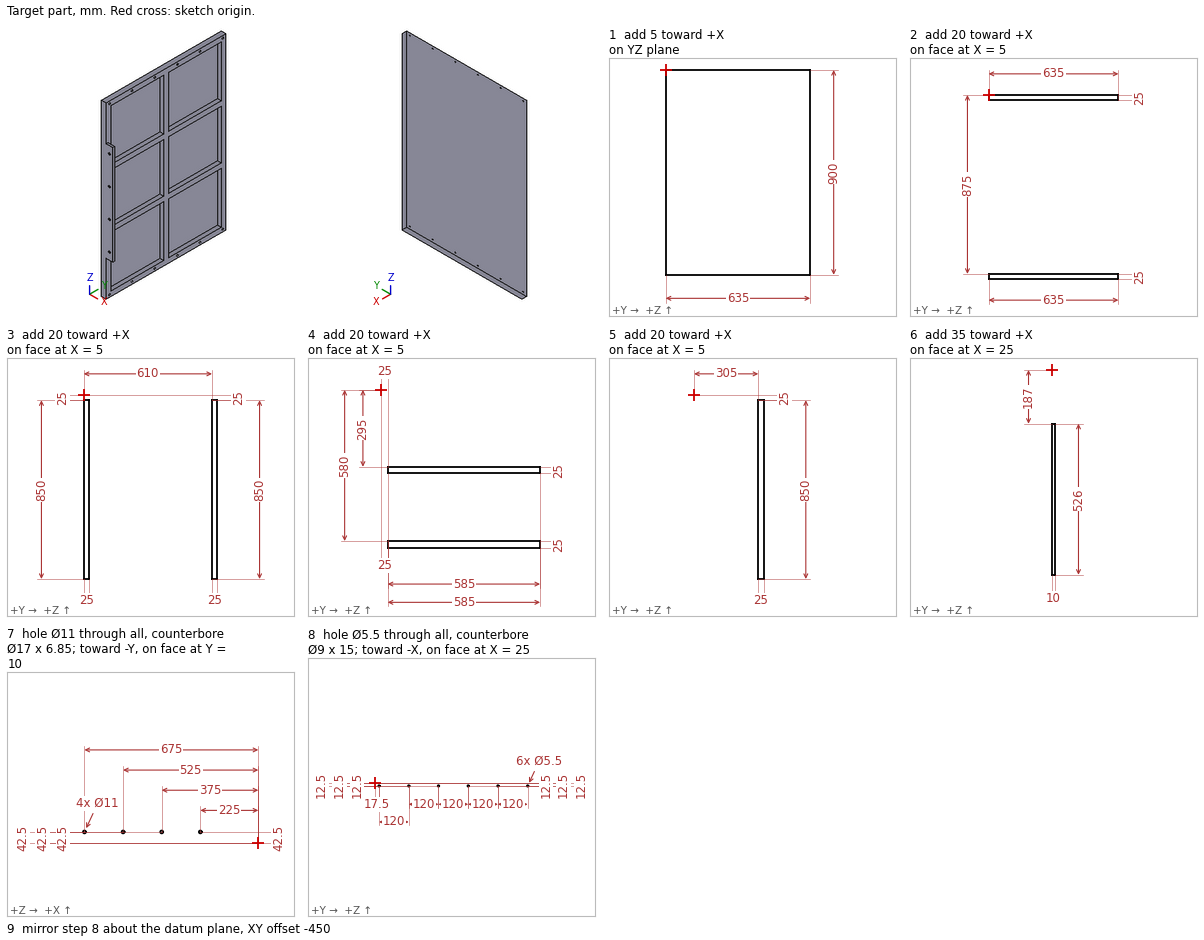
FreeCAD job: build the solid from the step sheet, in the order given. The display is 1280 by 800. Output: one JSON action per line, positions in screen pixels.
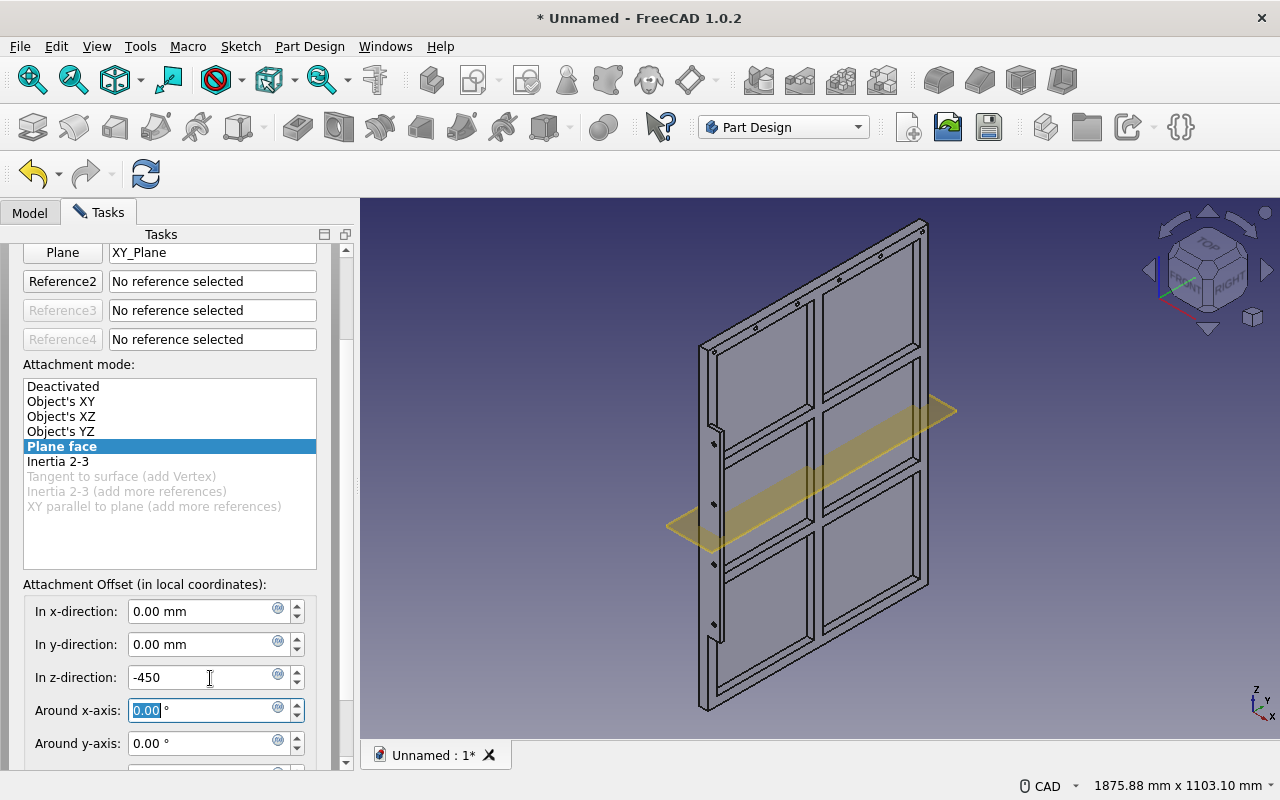
{"action": "scroll", "coordinate": [346, 507], "scroll_direction": "up", "scroll_amount": 3}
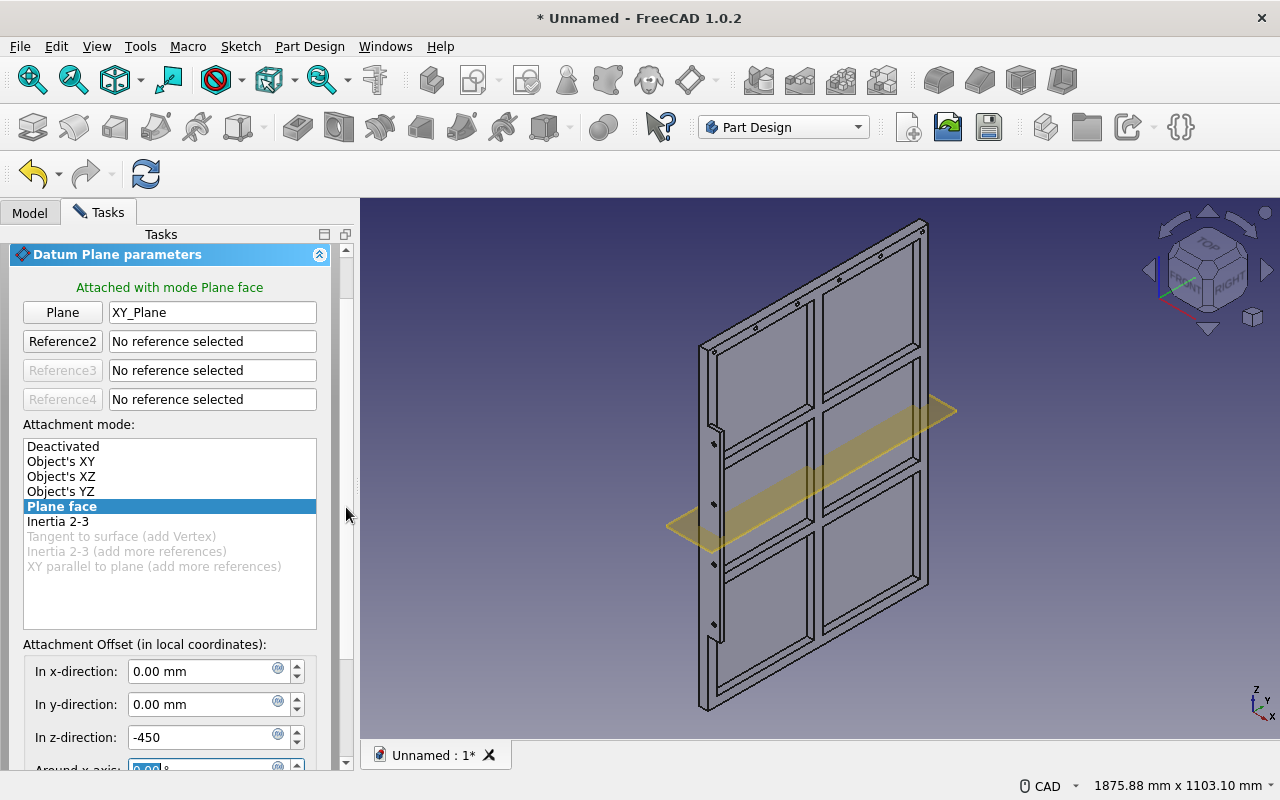
{"action": "left_click", "coordinate": [127, 273]}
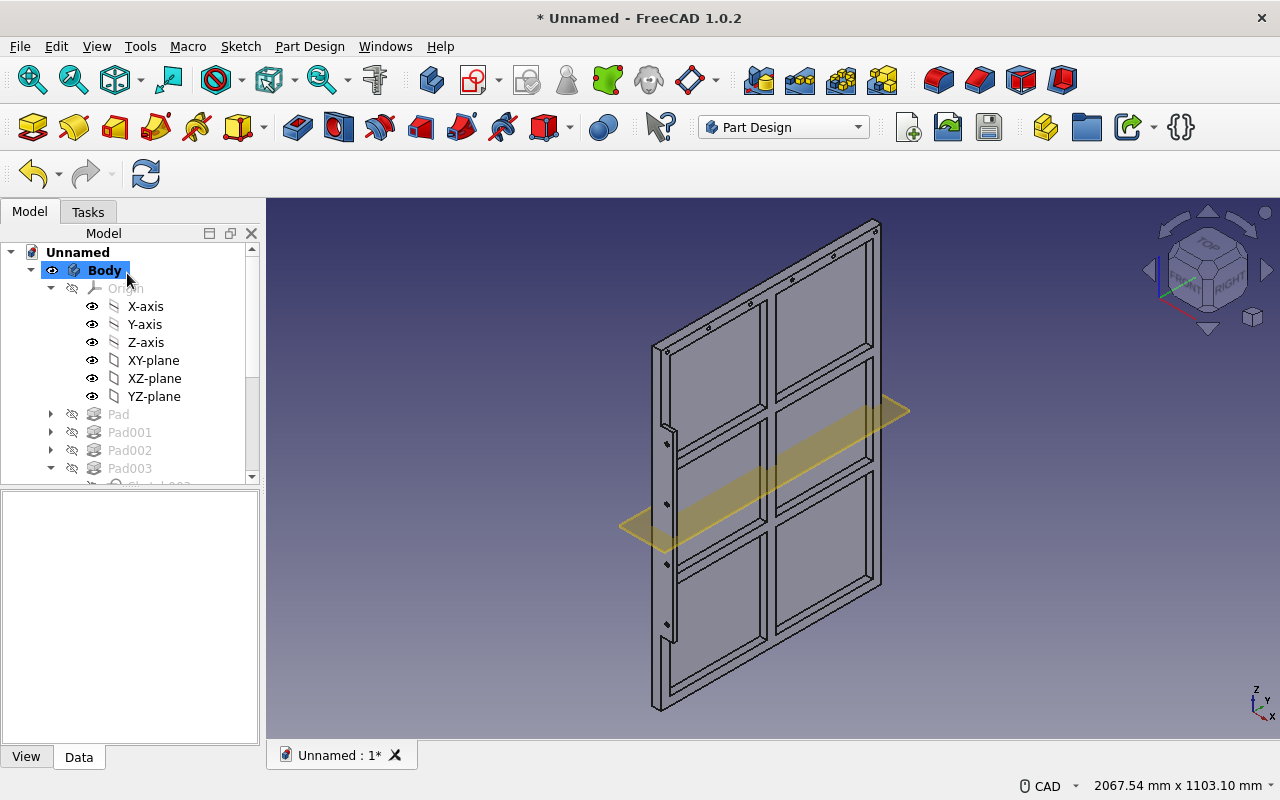
{"action": "scroll", "coordinate": [101, 356], "scroll_direction": "down", "scroll_amount": 3}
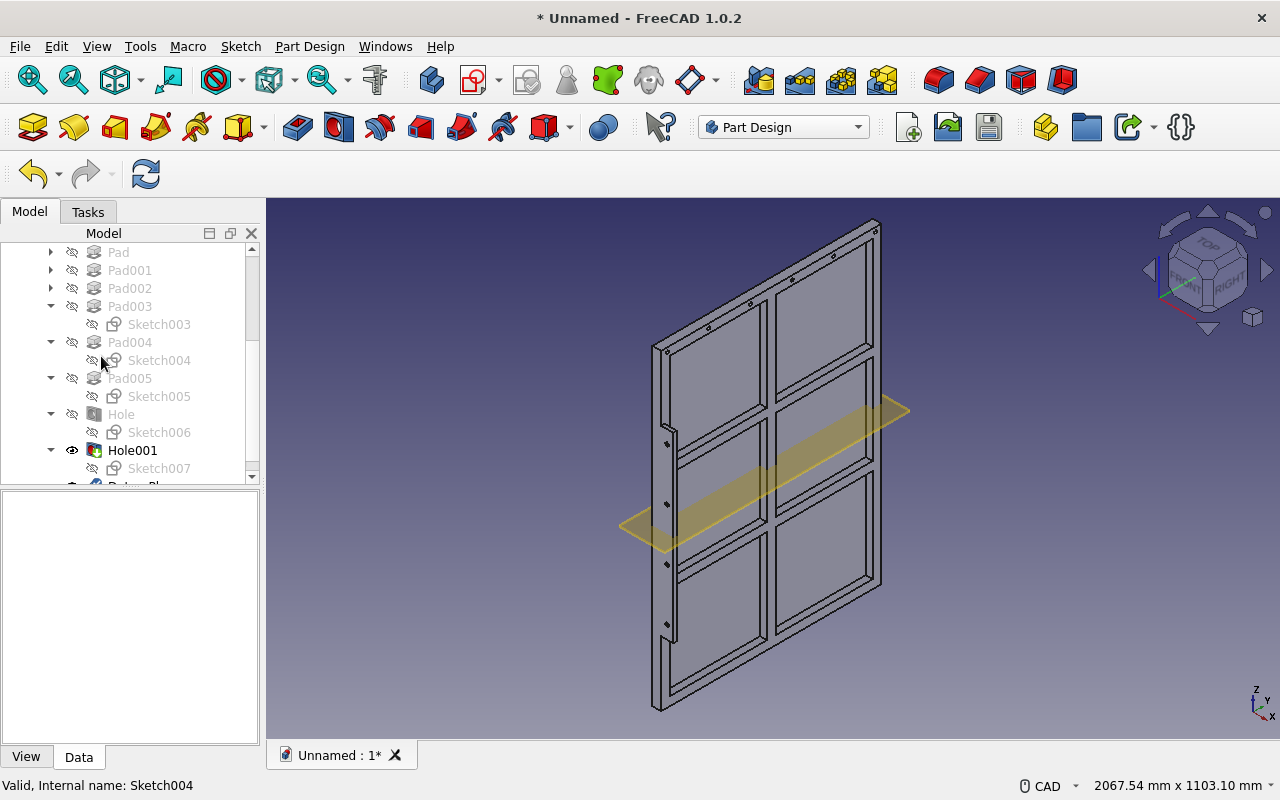
{"action": "left_click", "coordinate": [117, 450]}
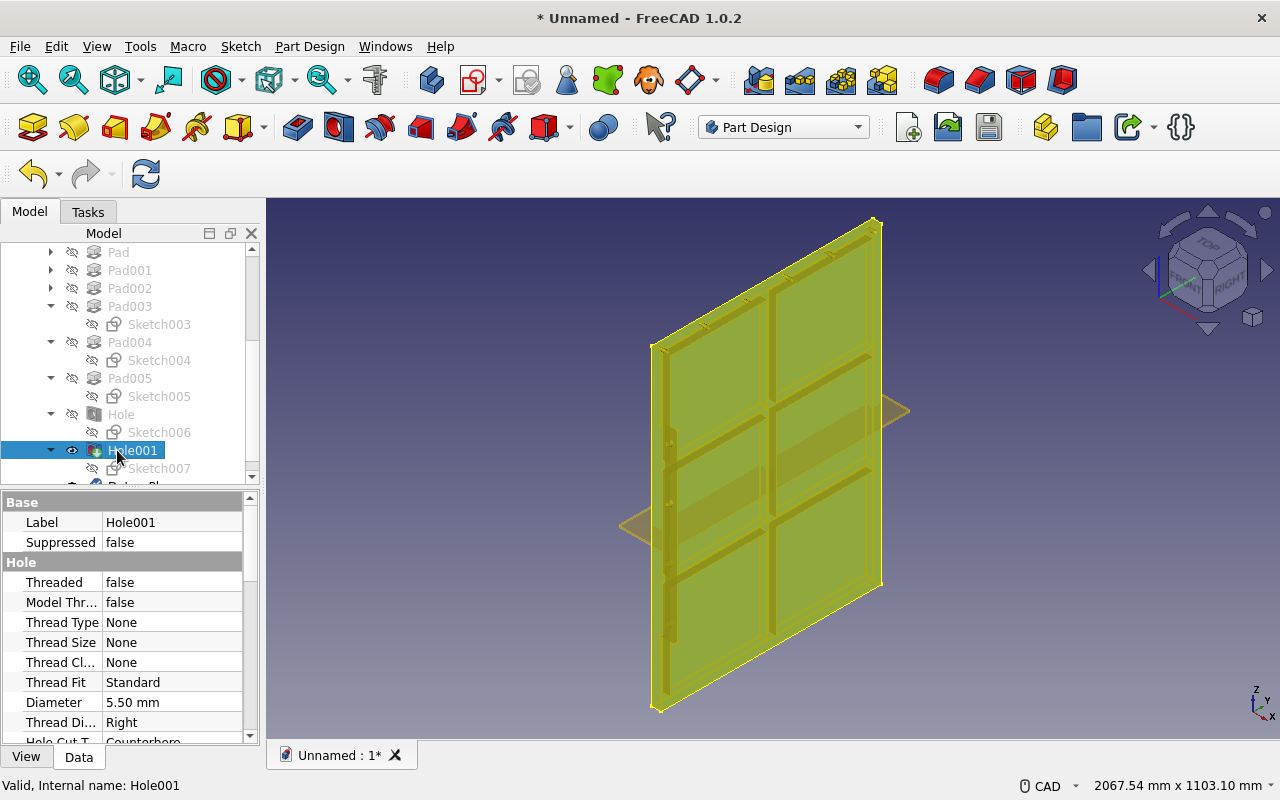
{"action": "left_click", "coordinate": [759, 80]}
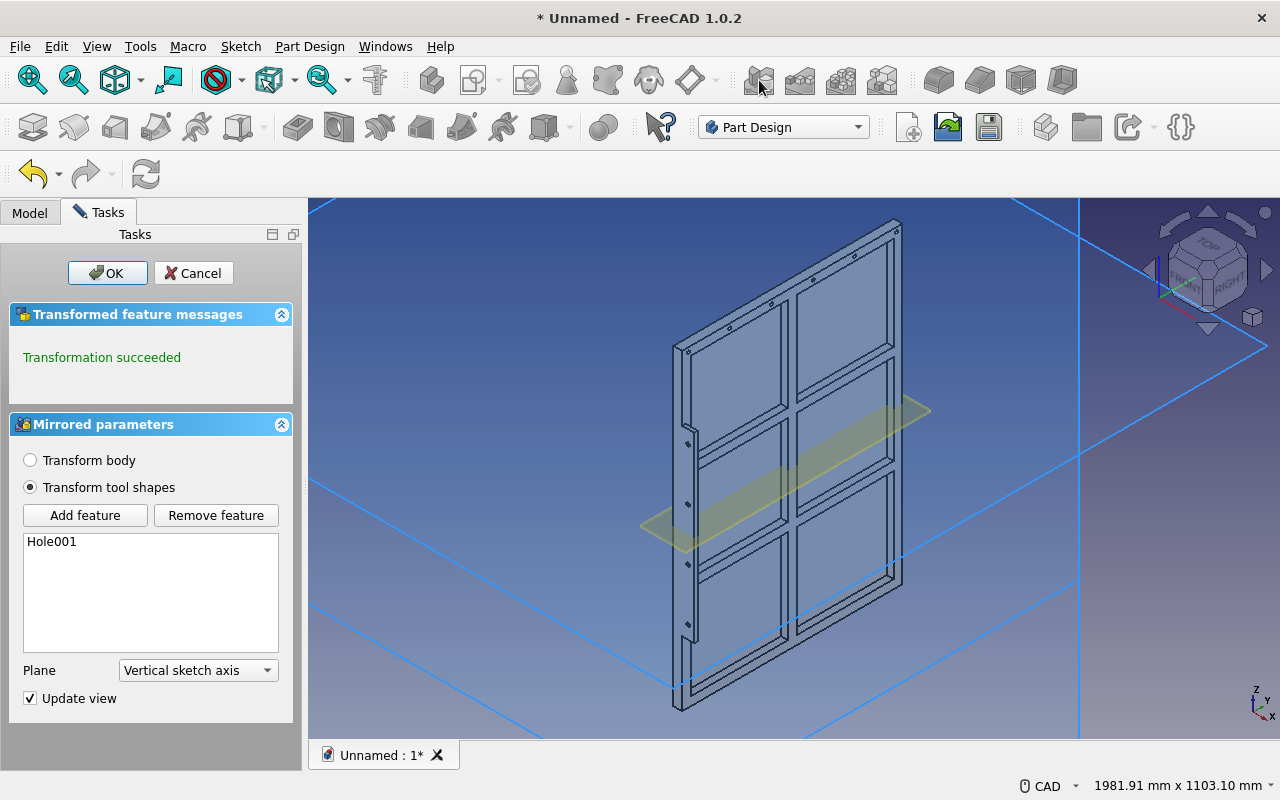
{"action": "left_click", "coordinate": [199, 670]}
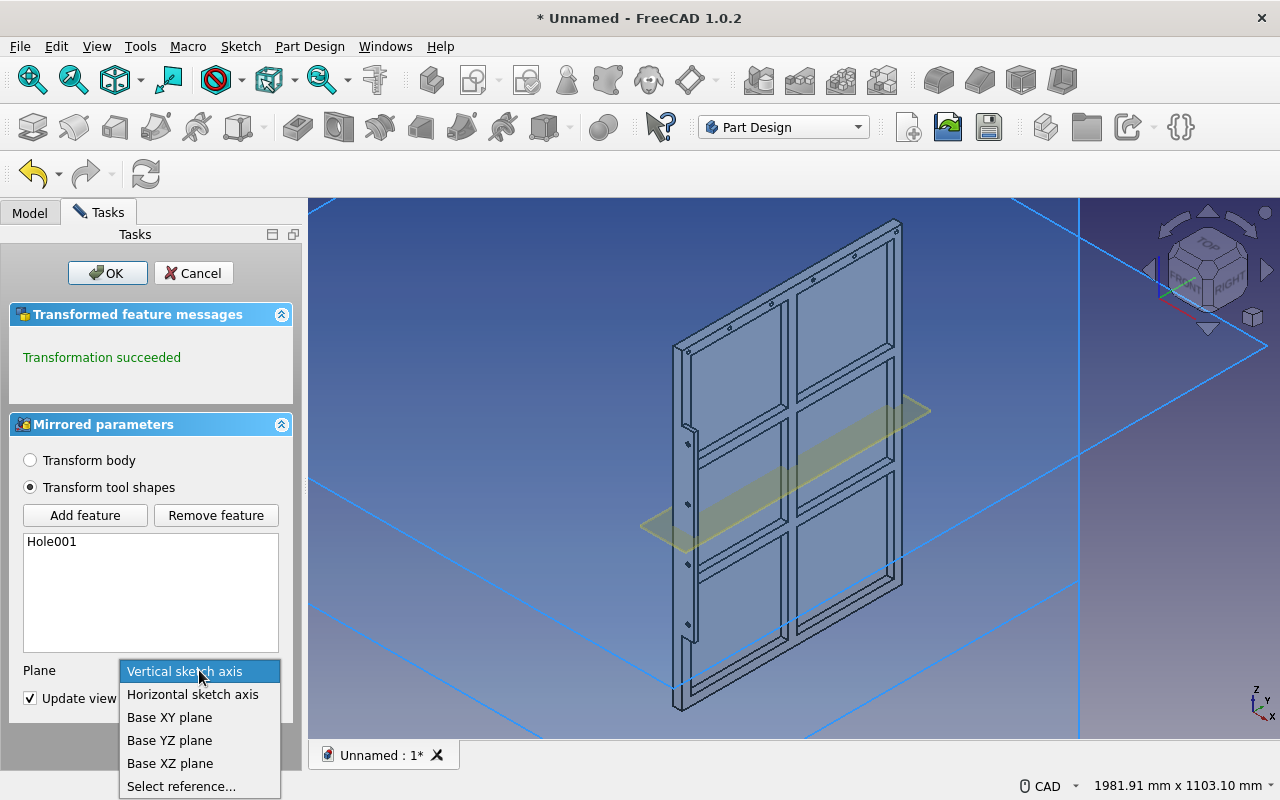
{"action": "left_click", "coordinate": [198, 786]}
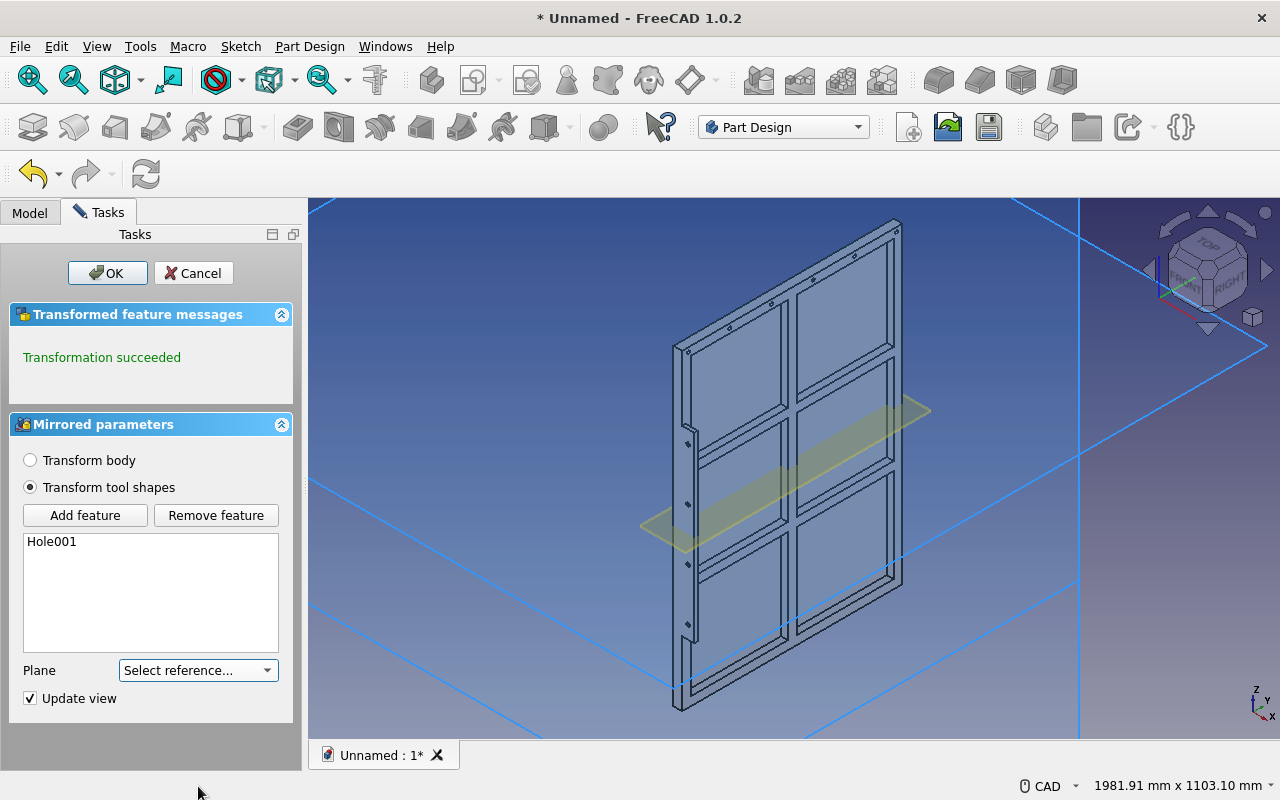
{"action": "left_click", "coordinate": [30, 212]}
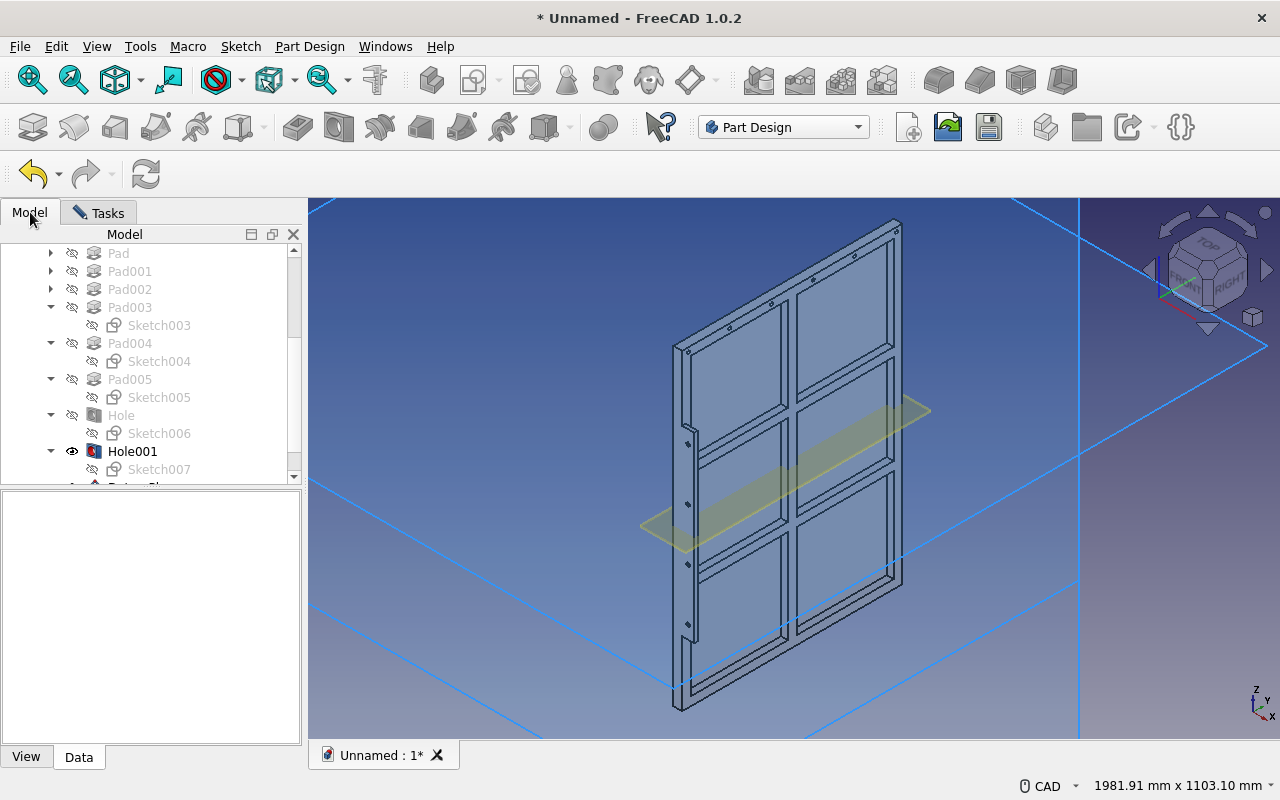
{"action": "scroll", "coordinate": [141, 357], "scroll_direction": "down", "scroll_amount": 3}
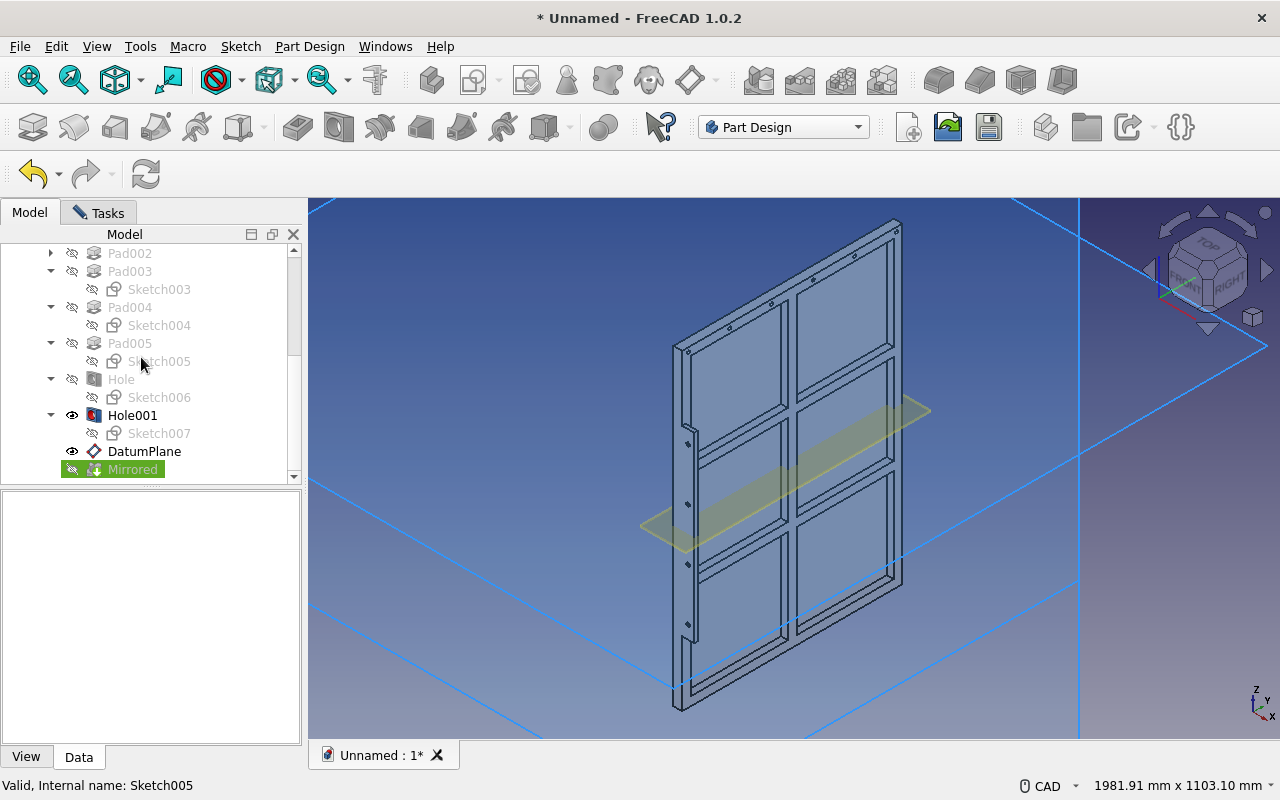
{"action": "left_click", "coordinate": [117, 451]}